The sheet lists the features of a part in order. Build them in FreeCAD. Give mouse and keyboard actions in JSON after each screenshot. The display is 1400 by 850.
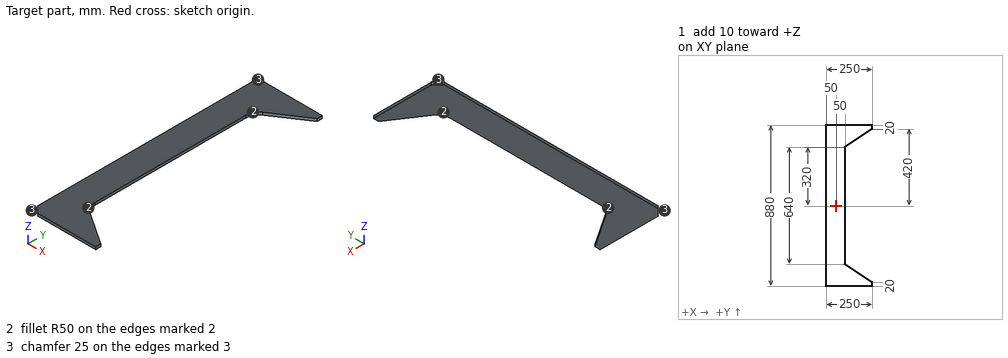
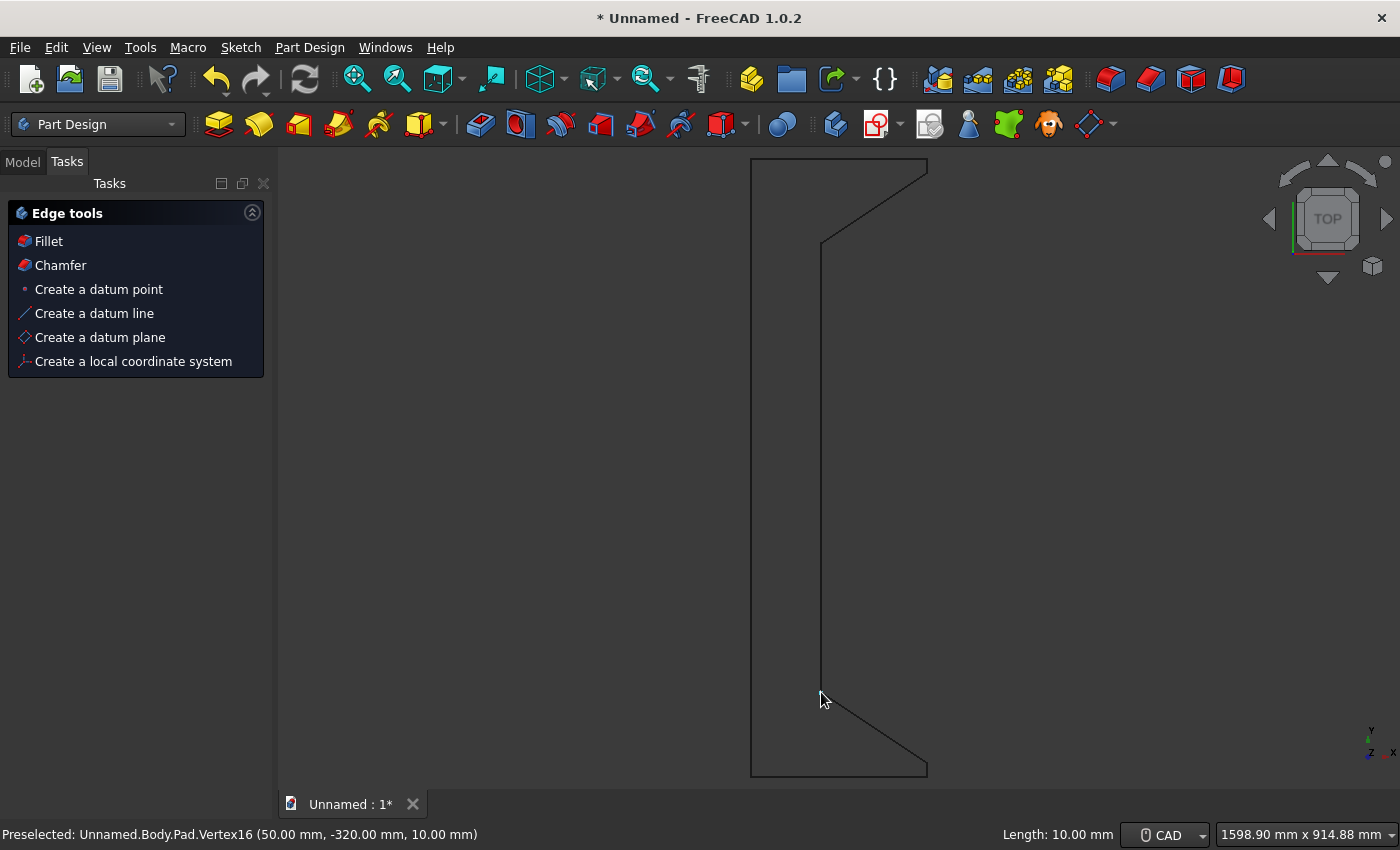
{"action": "key", "text": "1"}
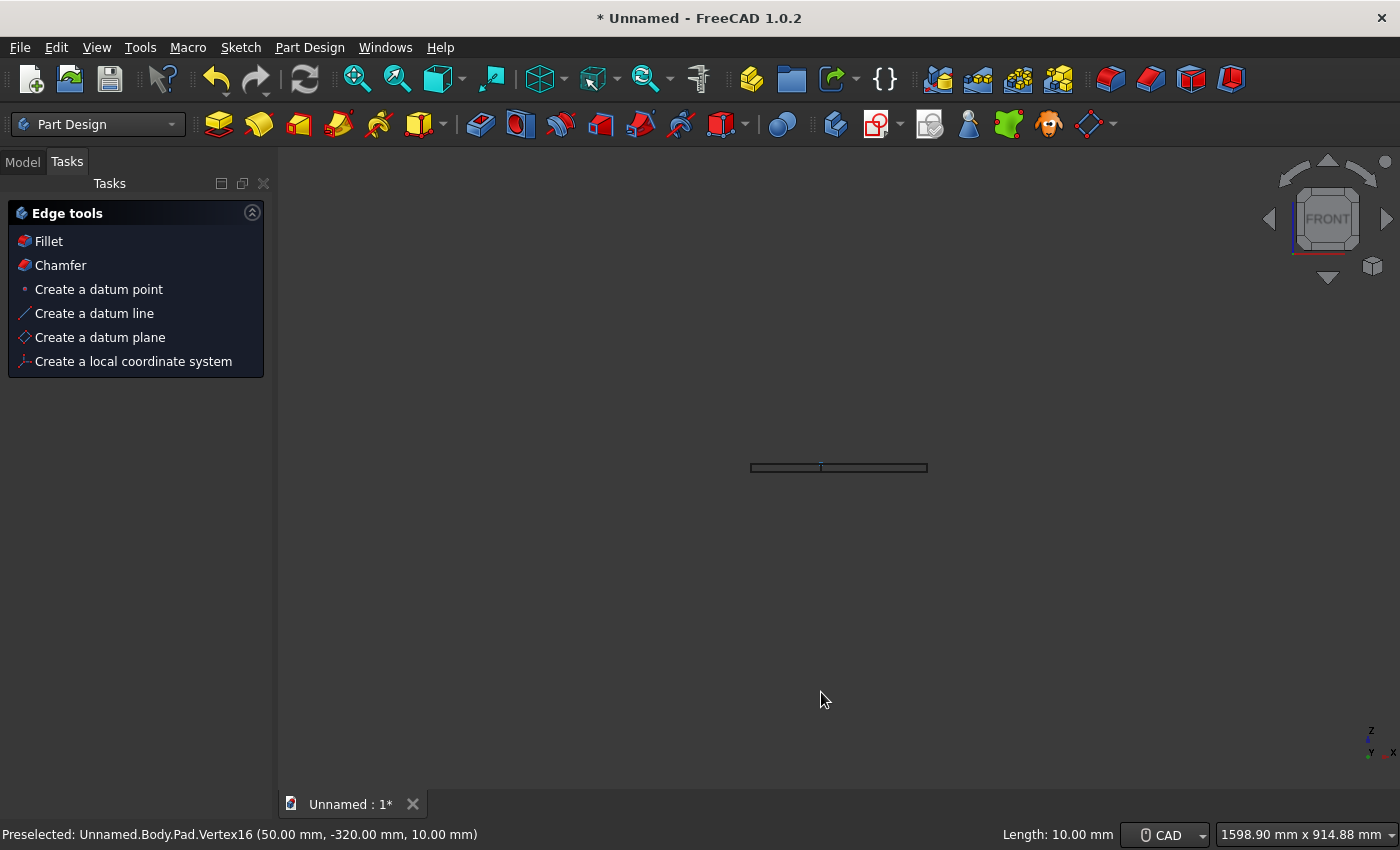
{"action": "left_click", "coordinate": [358, 80]}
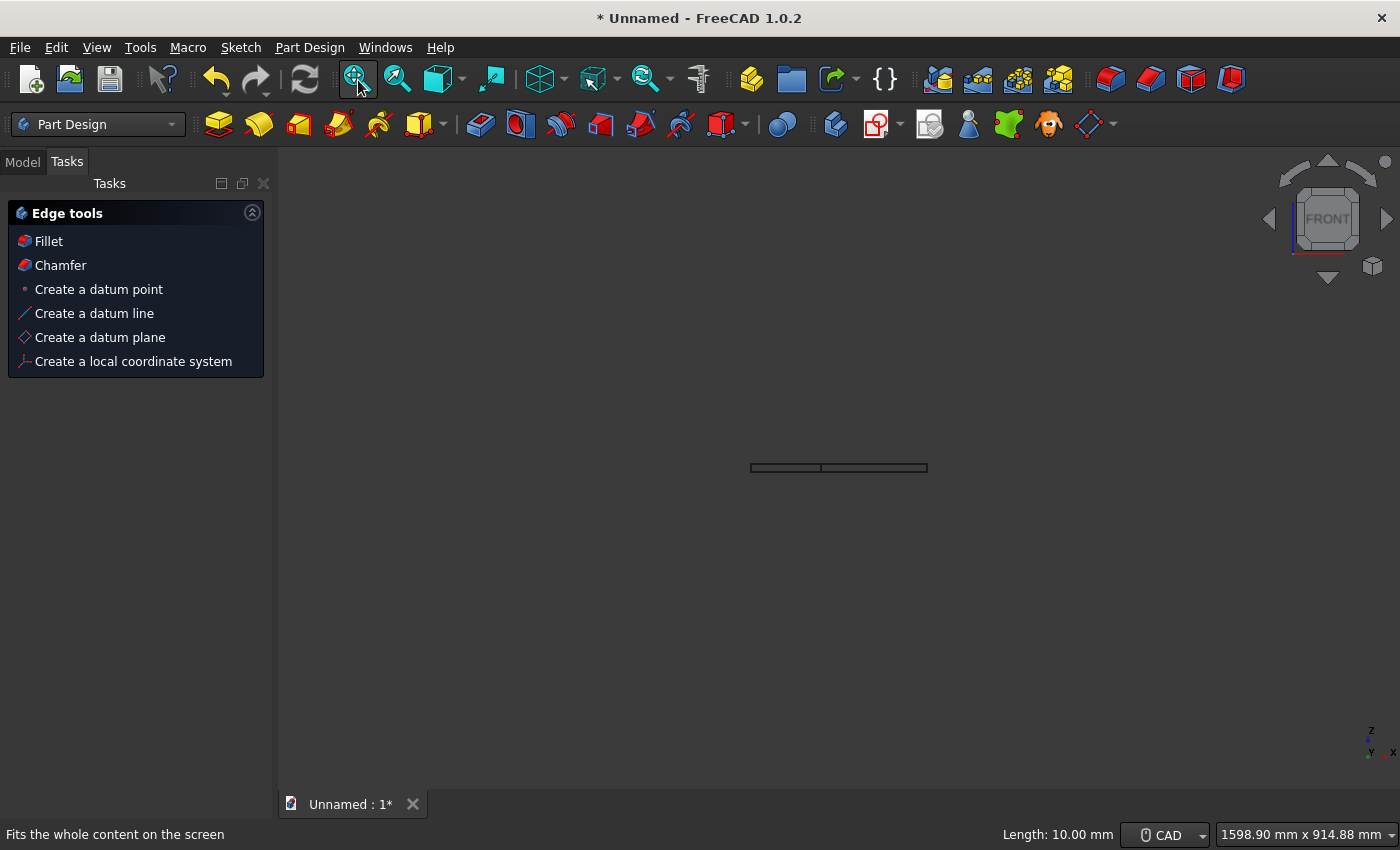
{"action": "scroll", "coordinate": [821, 467], "scroll_direction": "up", "scroll_amount": 9}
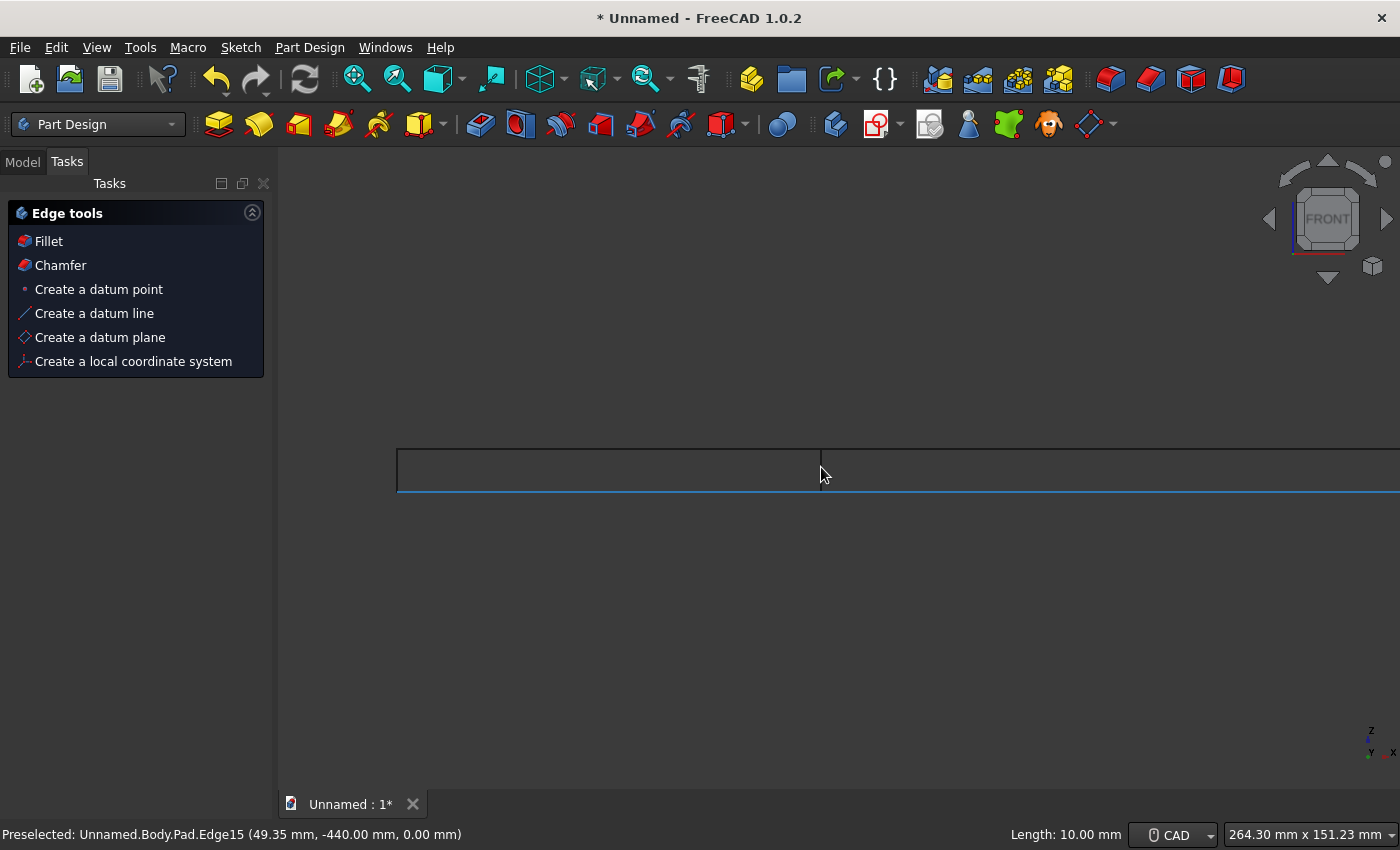
{"action": "left_click", "coordinate": [821, 470], "text": "ctrl"}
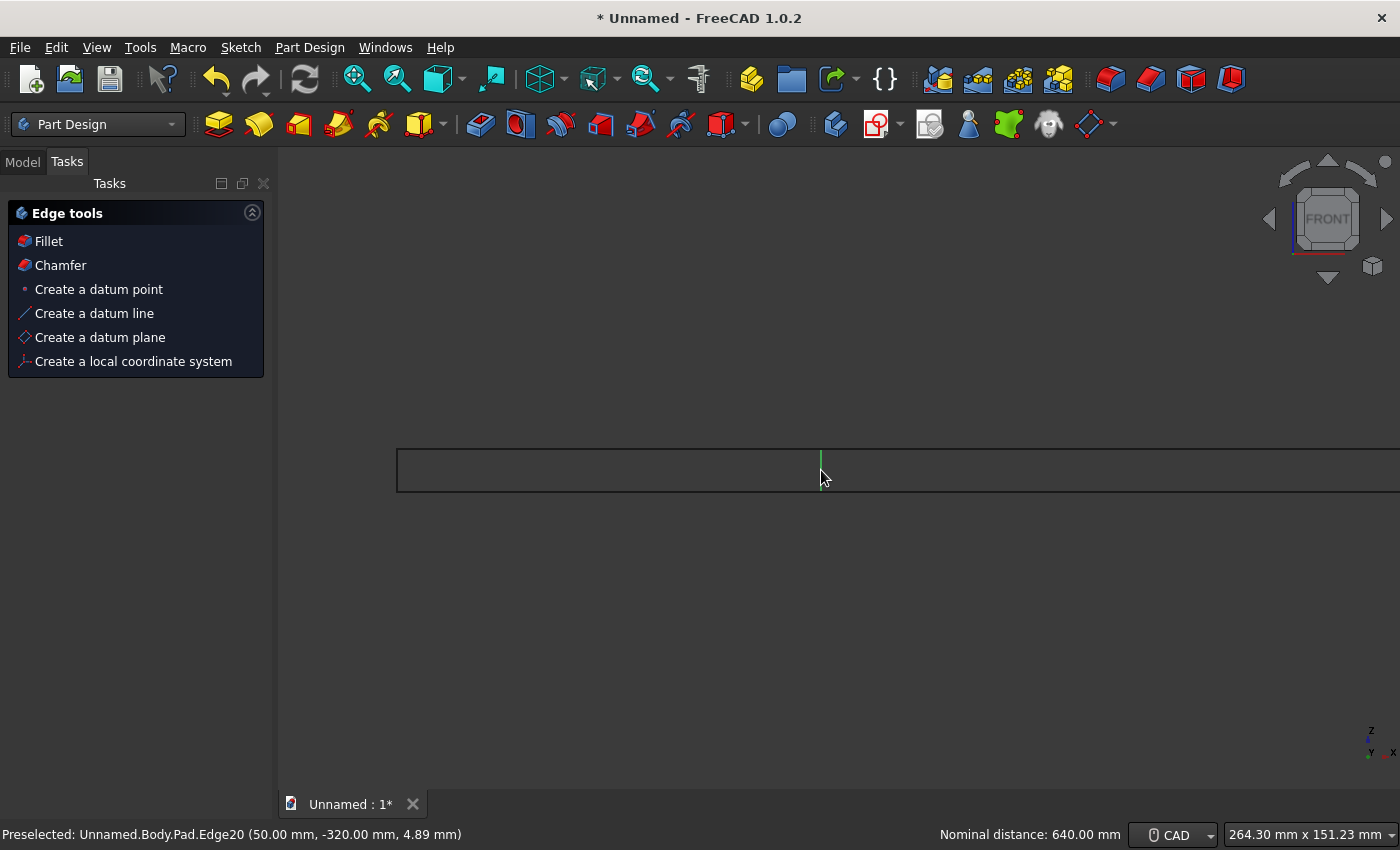
{"action": "key", "text": "v 1"}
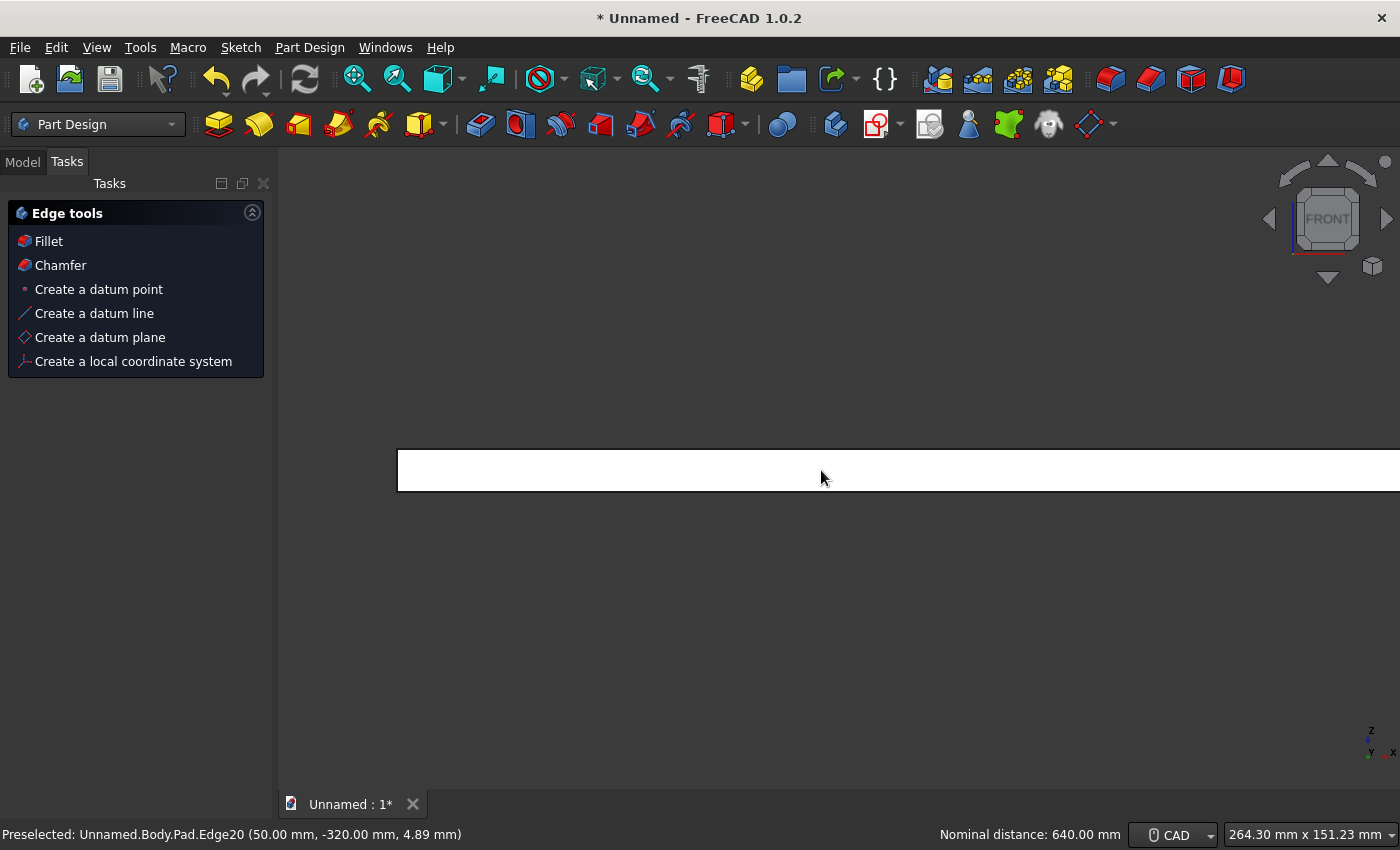
{"action": "left_click", "coordinate": [1112, 80]}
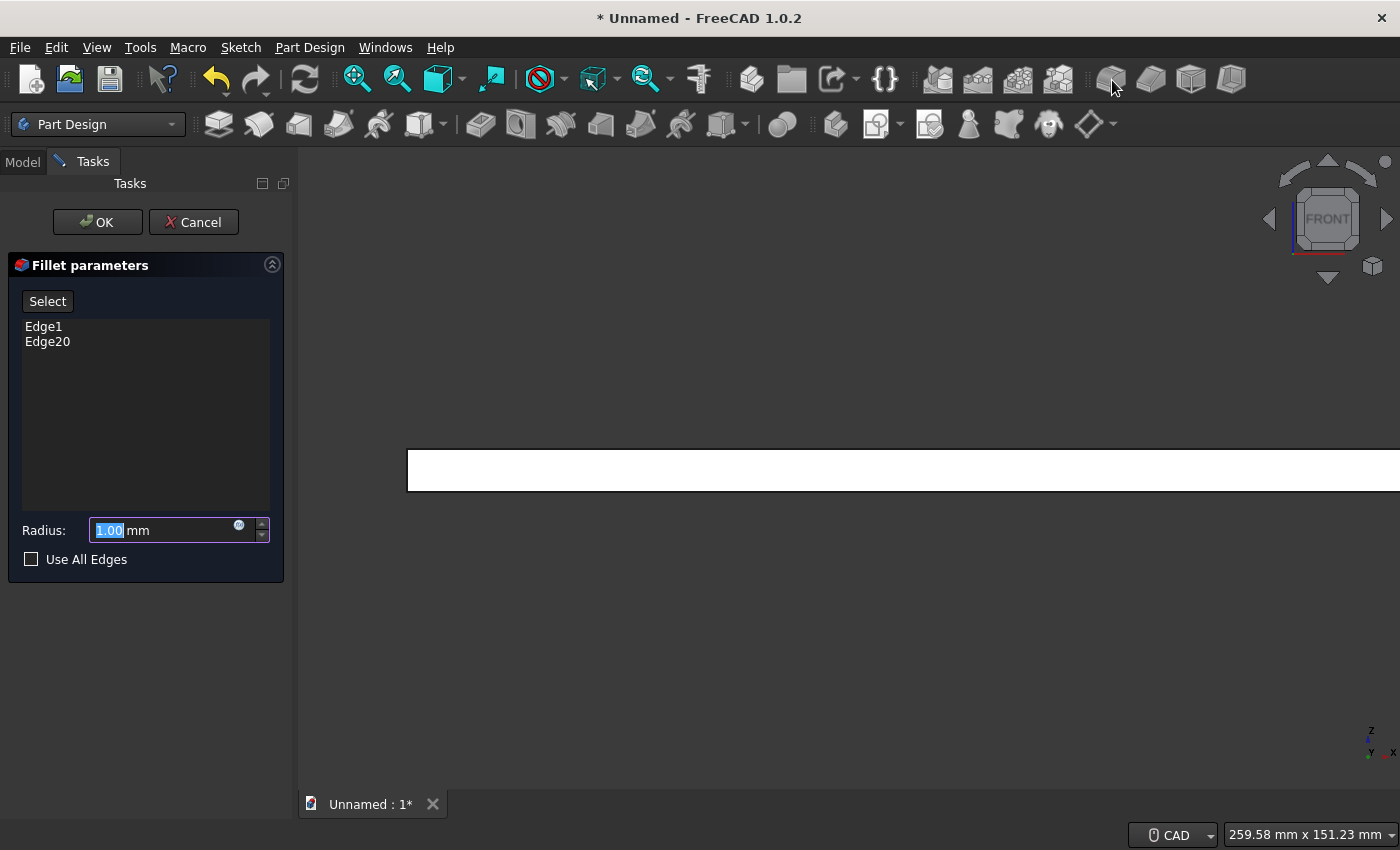
{"action": "type", "text": "50"}
{"action": "key", "text": "Tab"}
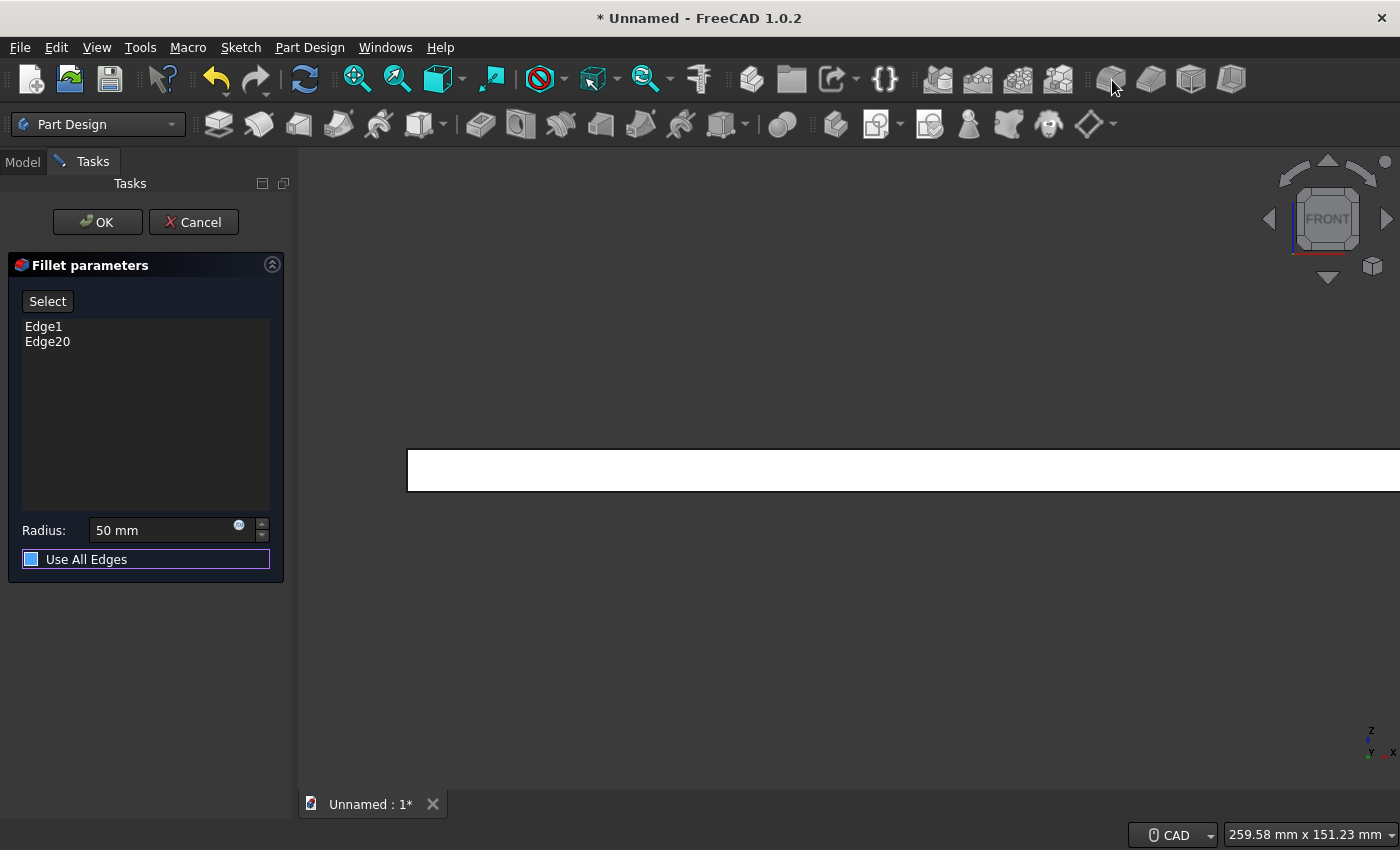
{"action": "left_click", "coordinate": [98, 222]}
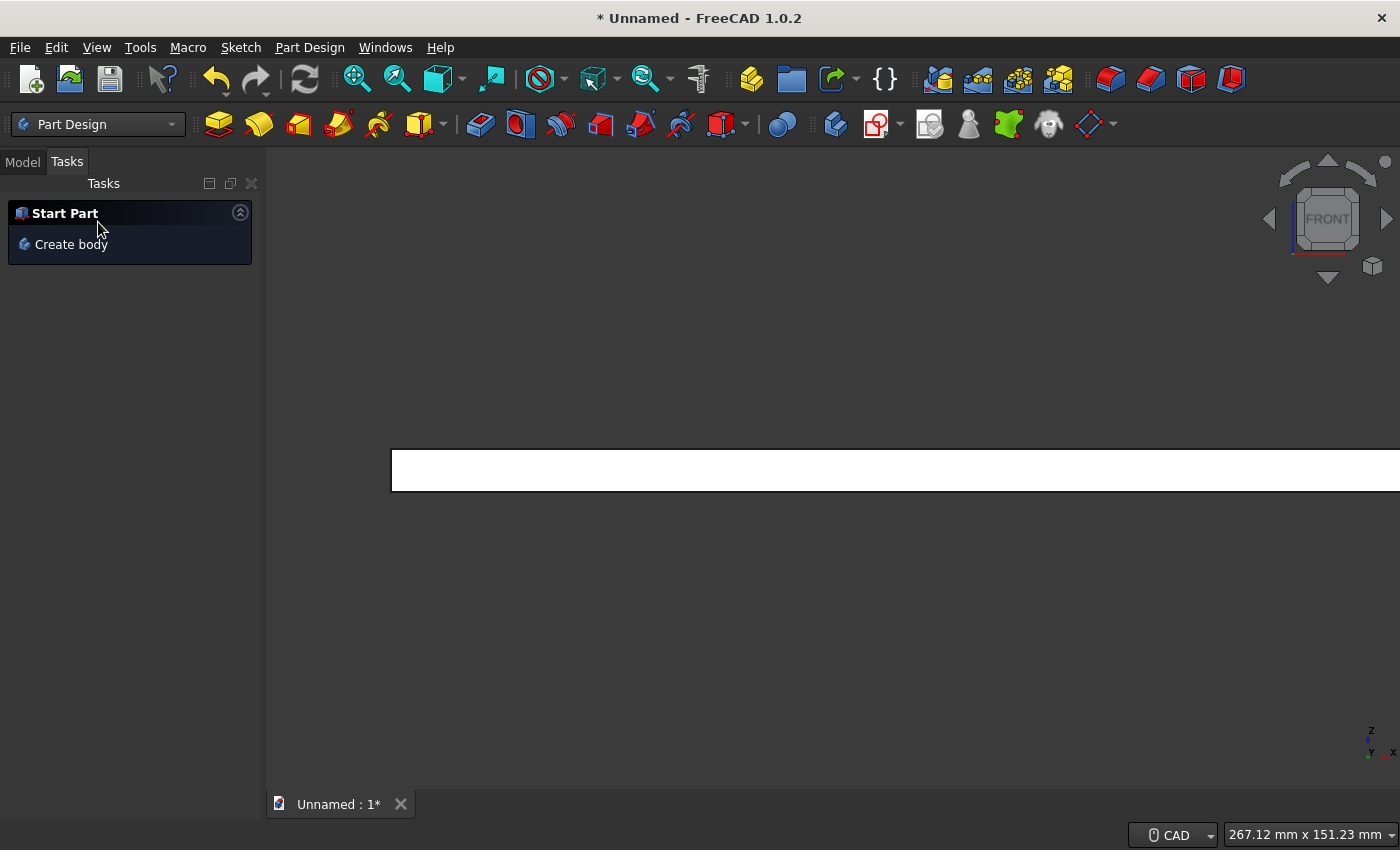
{"action": "key", "text": "v f"}